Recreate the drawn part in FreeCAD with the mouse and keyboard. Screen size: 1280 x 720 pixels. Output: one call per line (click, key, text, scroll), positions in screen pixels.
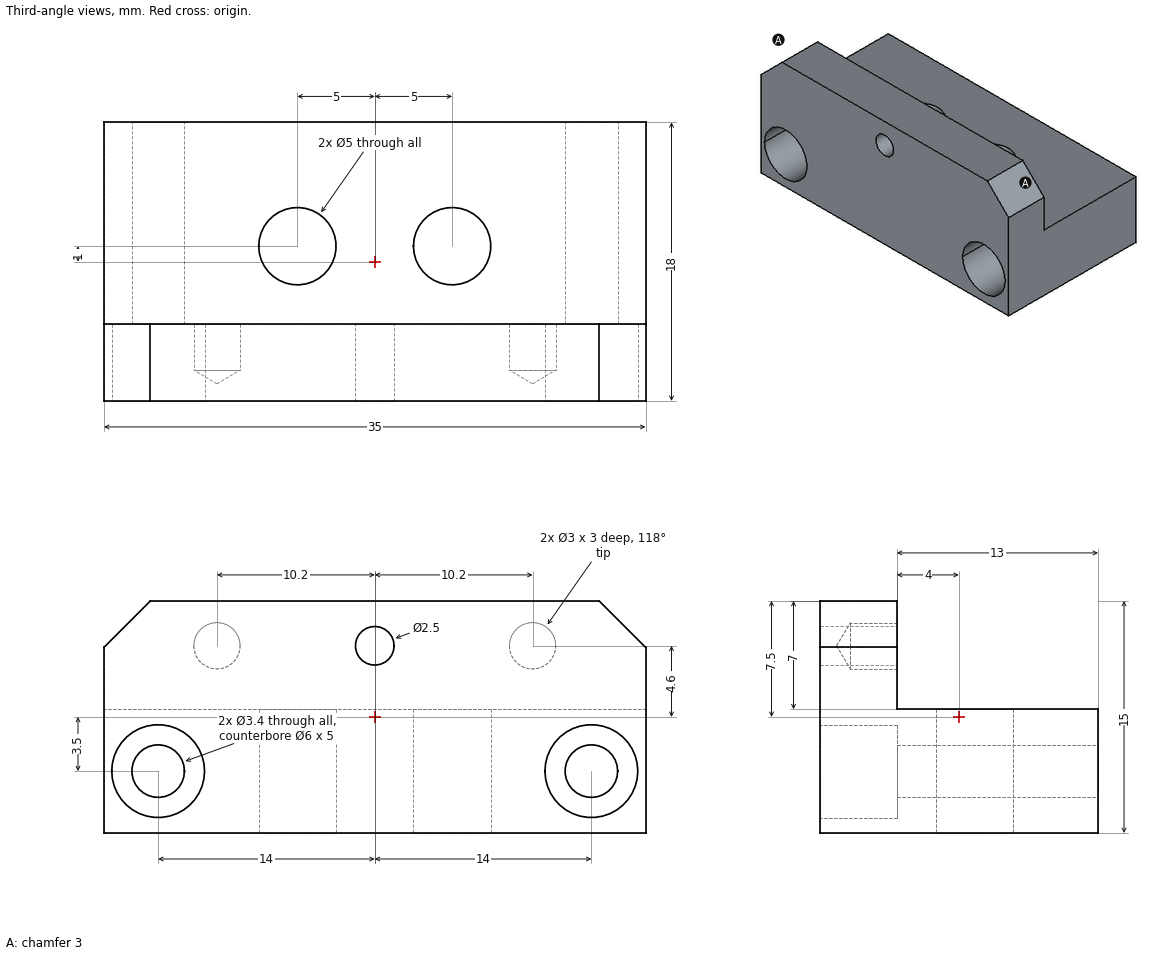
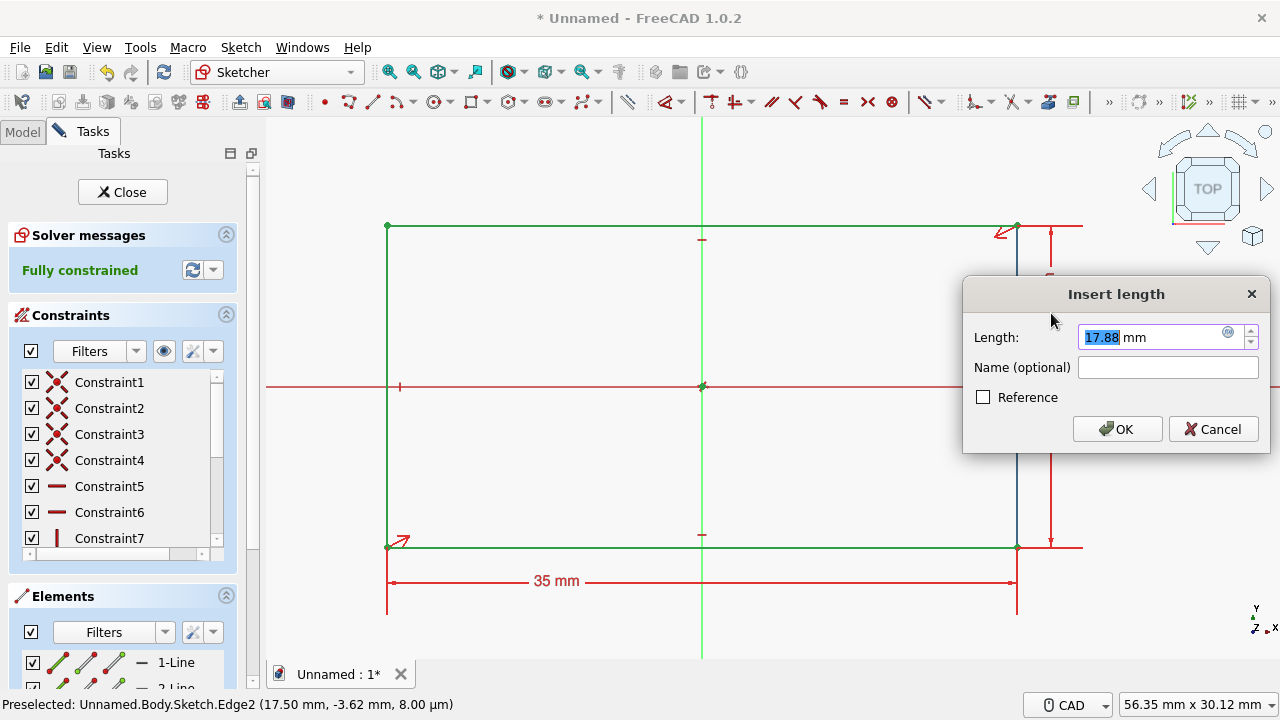
text(18)
key(Return)
key(Escape)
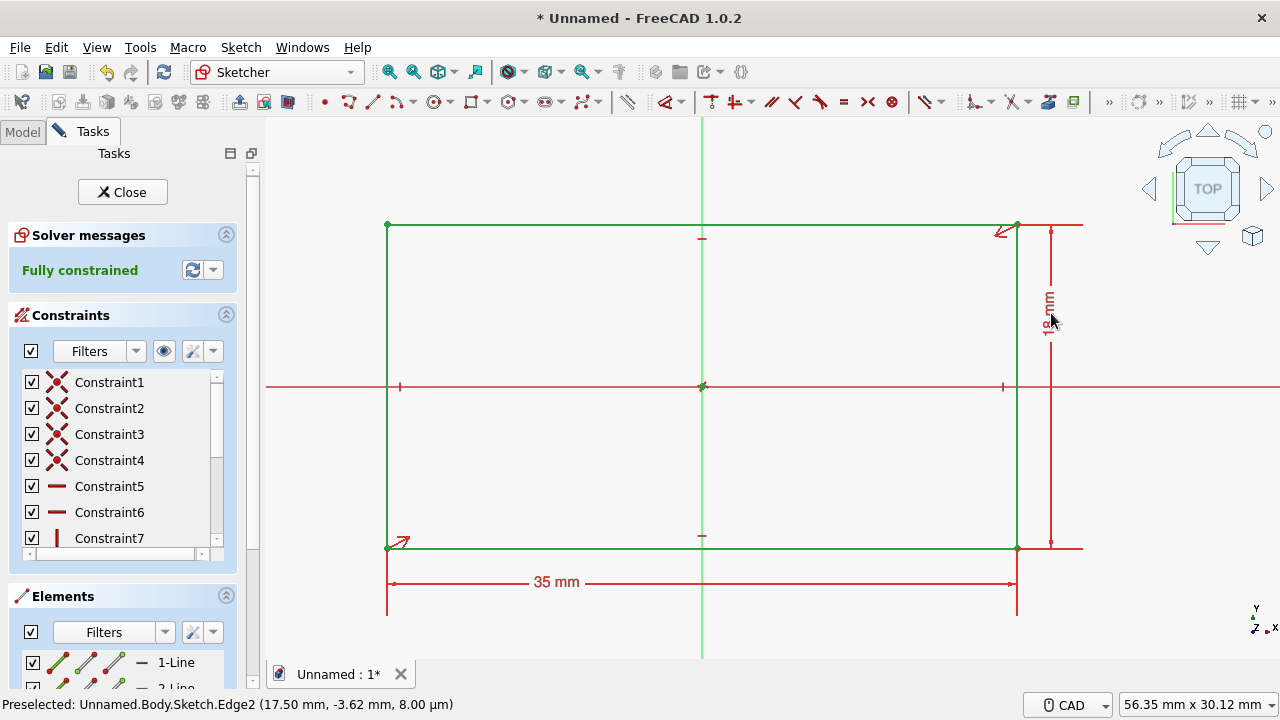
click(123, 192)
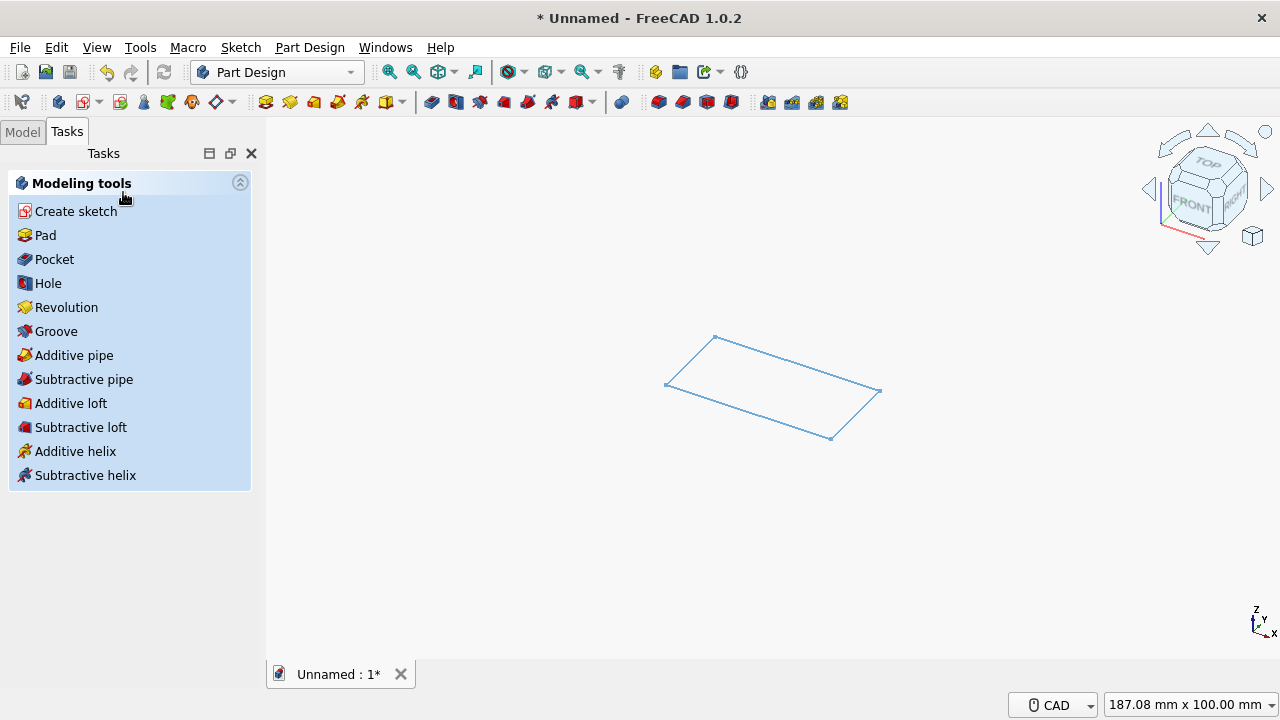
click(266, 102)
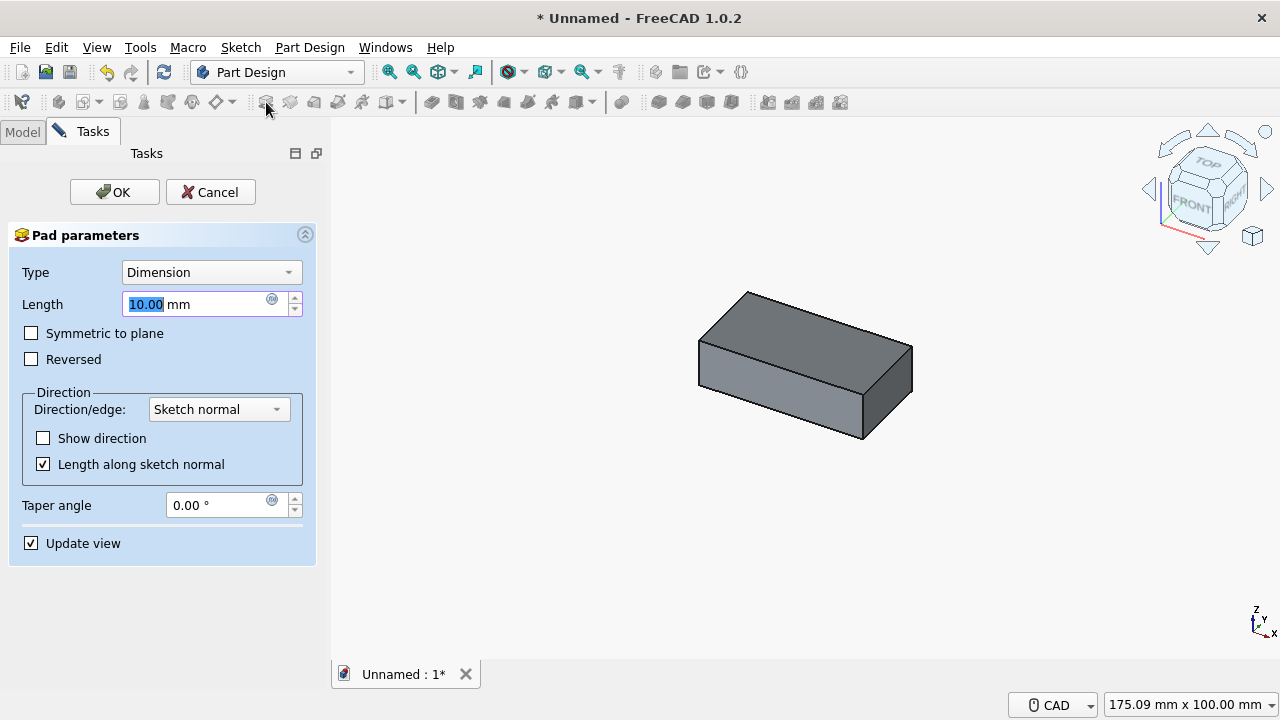
text(15)
key(Tab)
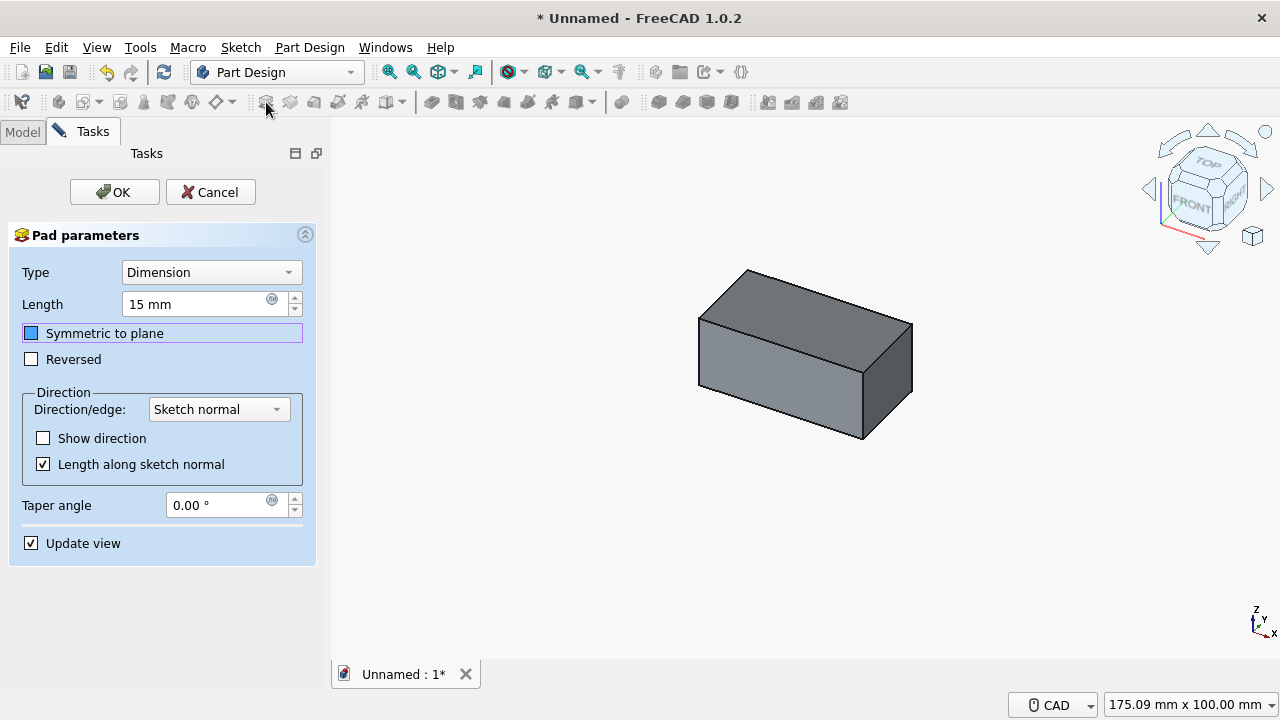
click(30, 333)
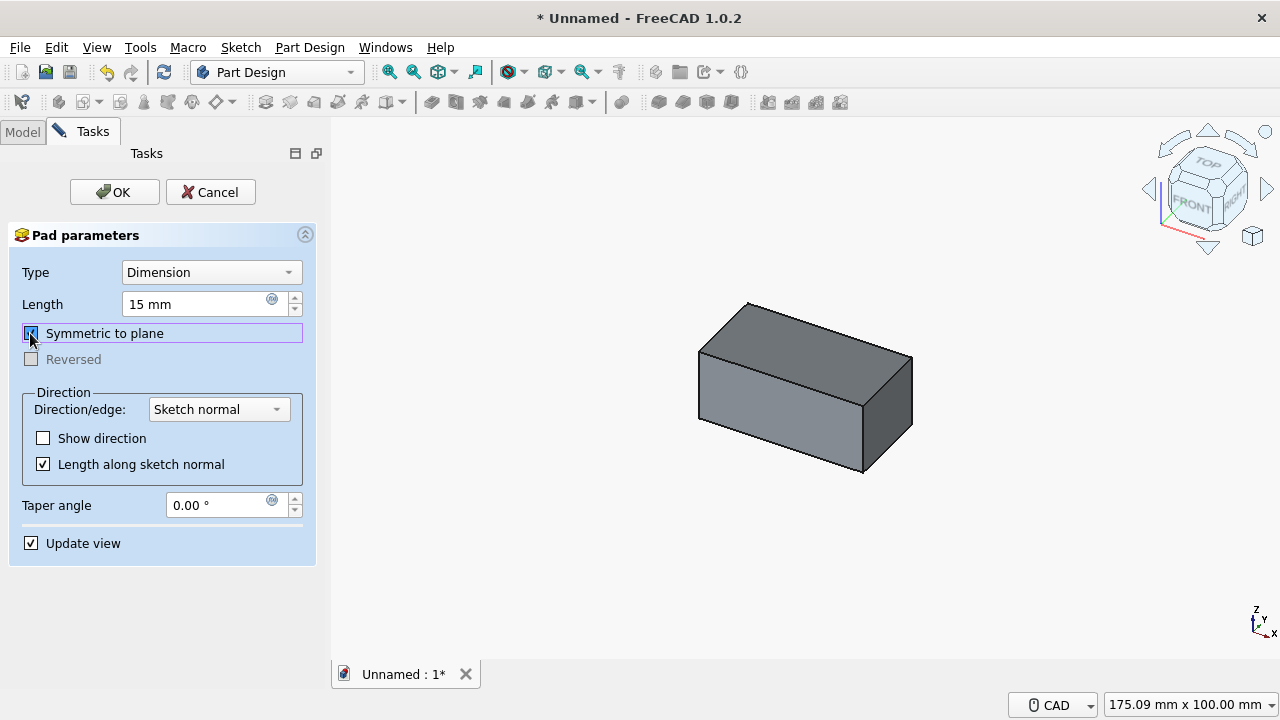
click(115, 192)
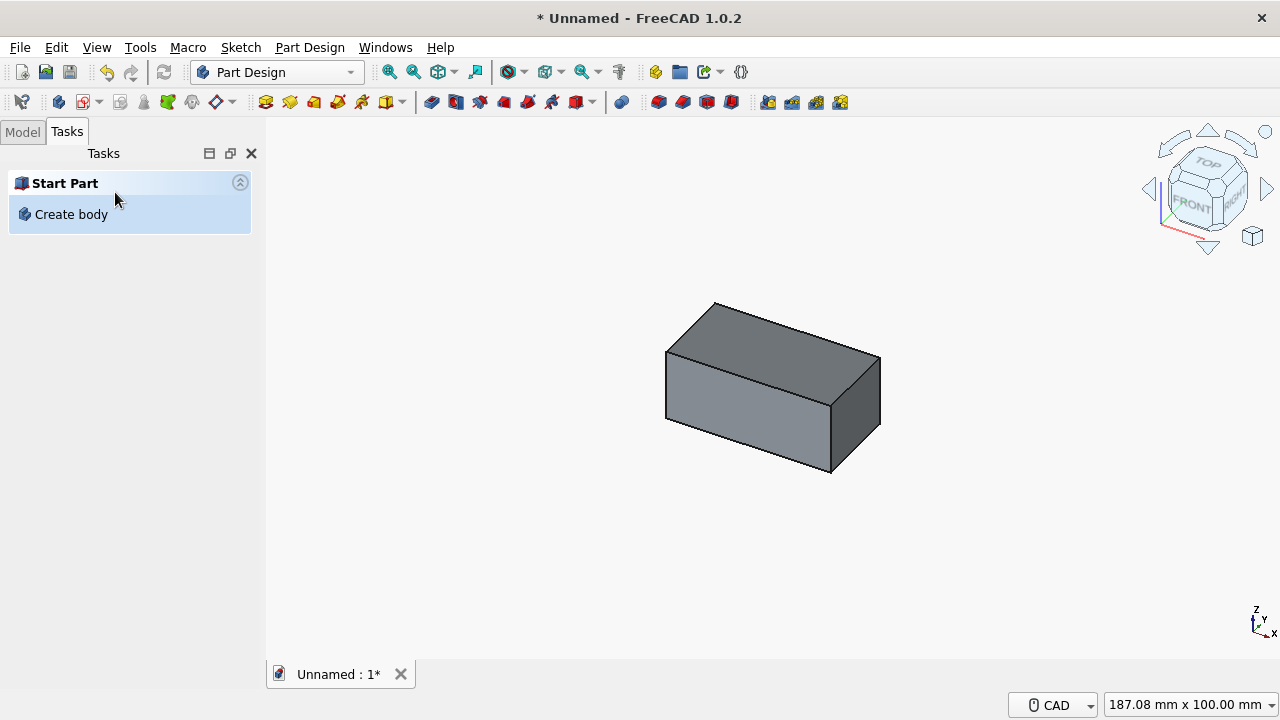
key(v)
key(f)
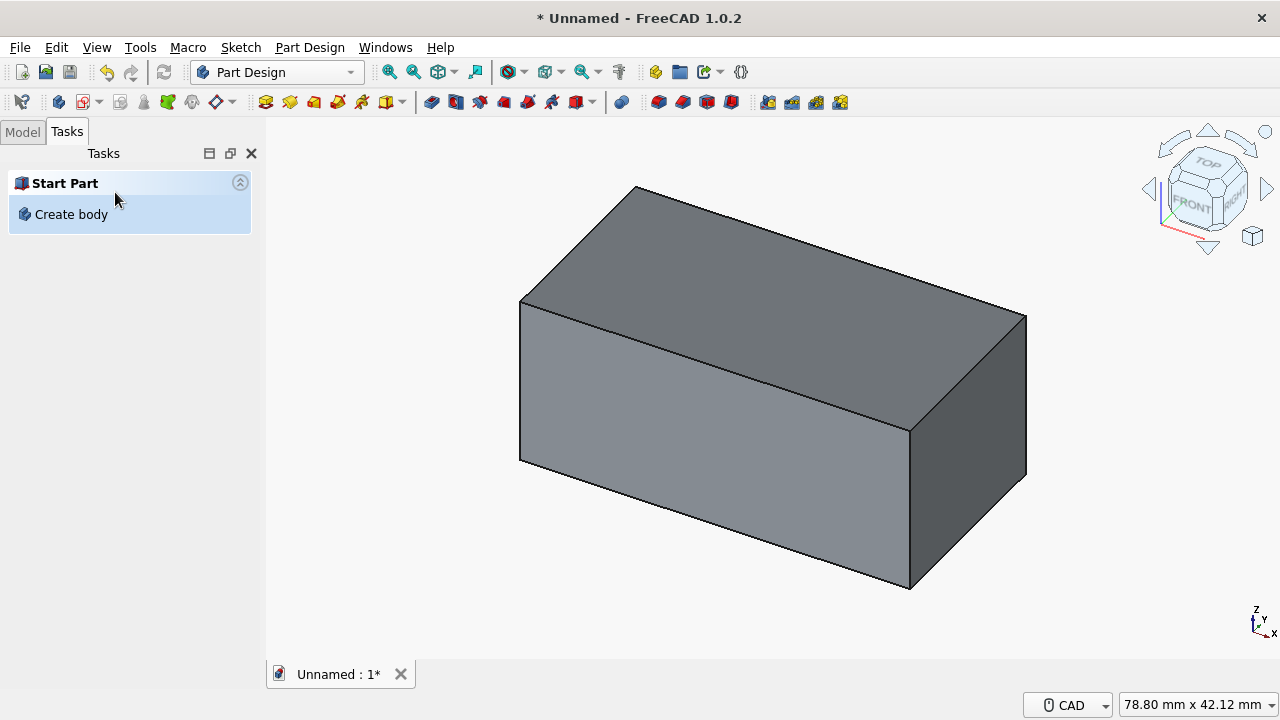
click(968, 452)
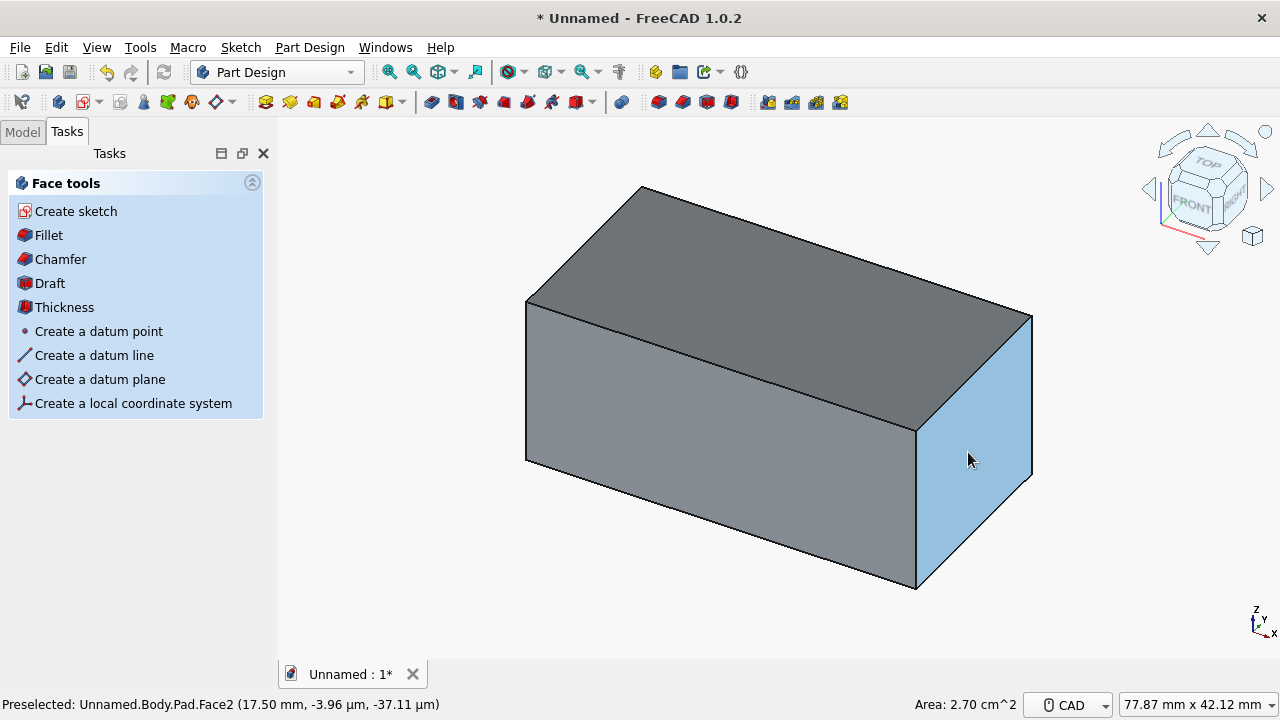
click(84, 102)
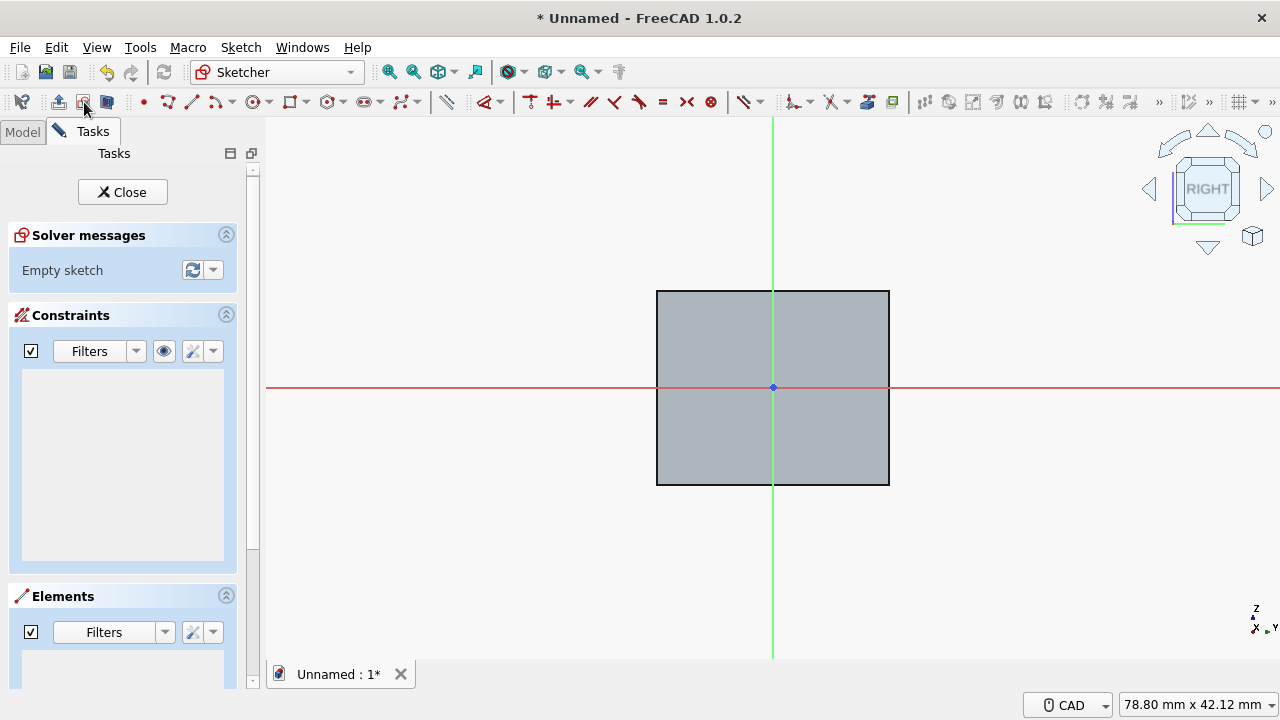
scroll(849, 319, up, 6)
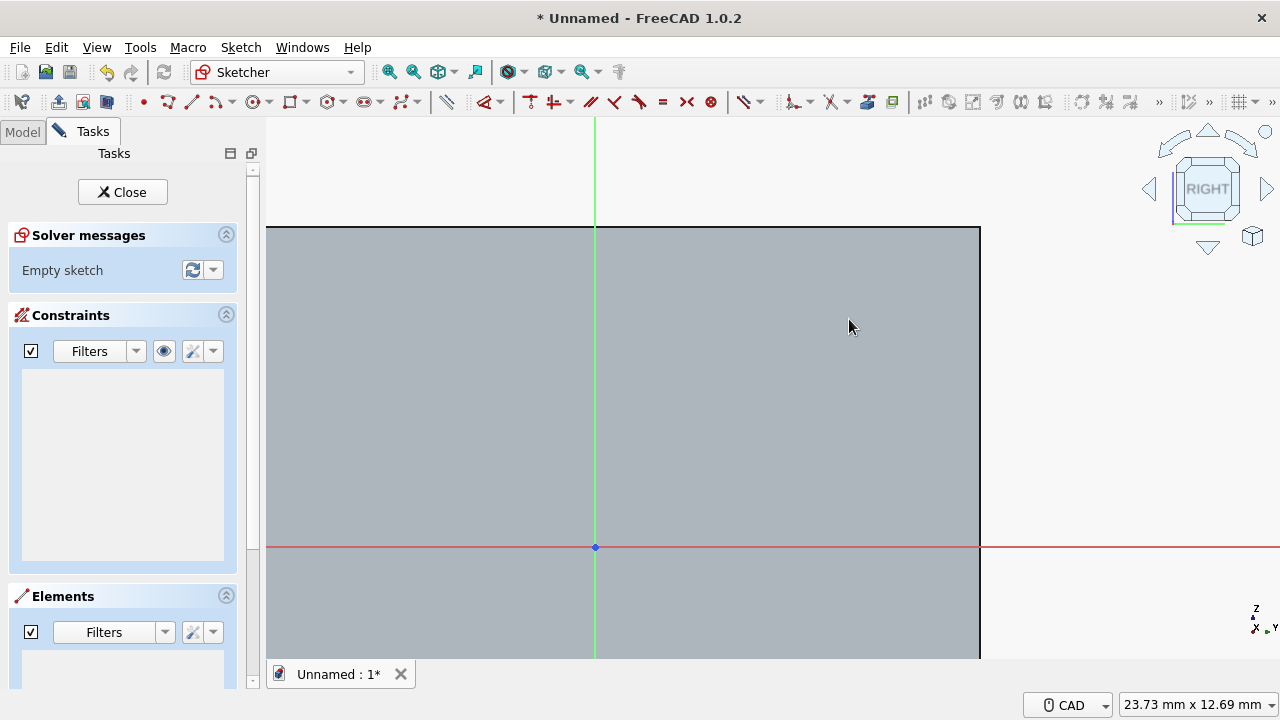
key(g)
key(r)